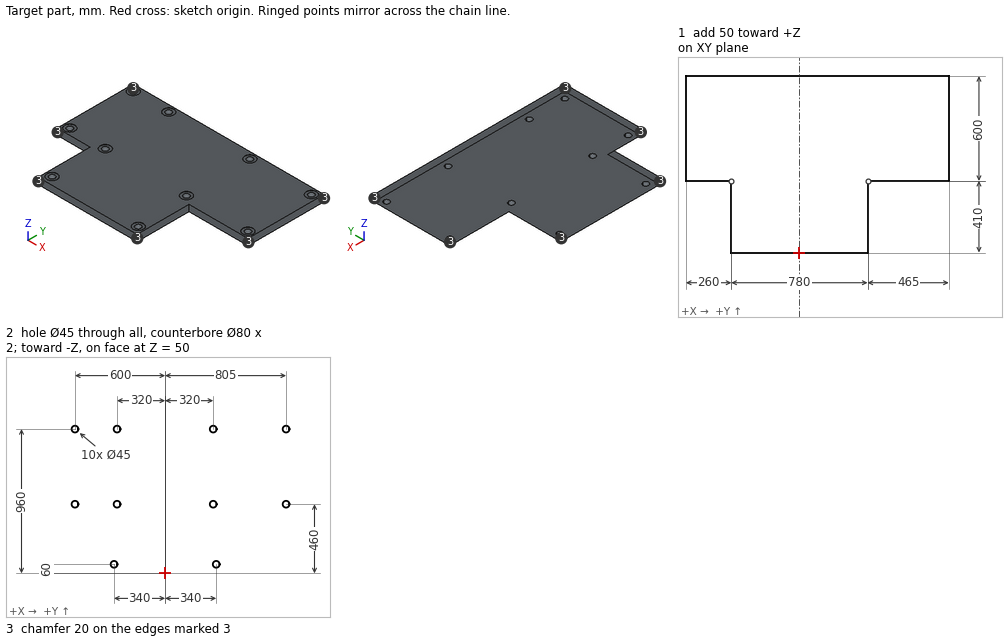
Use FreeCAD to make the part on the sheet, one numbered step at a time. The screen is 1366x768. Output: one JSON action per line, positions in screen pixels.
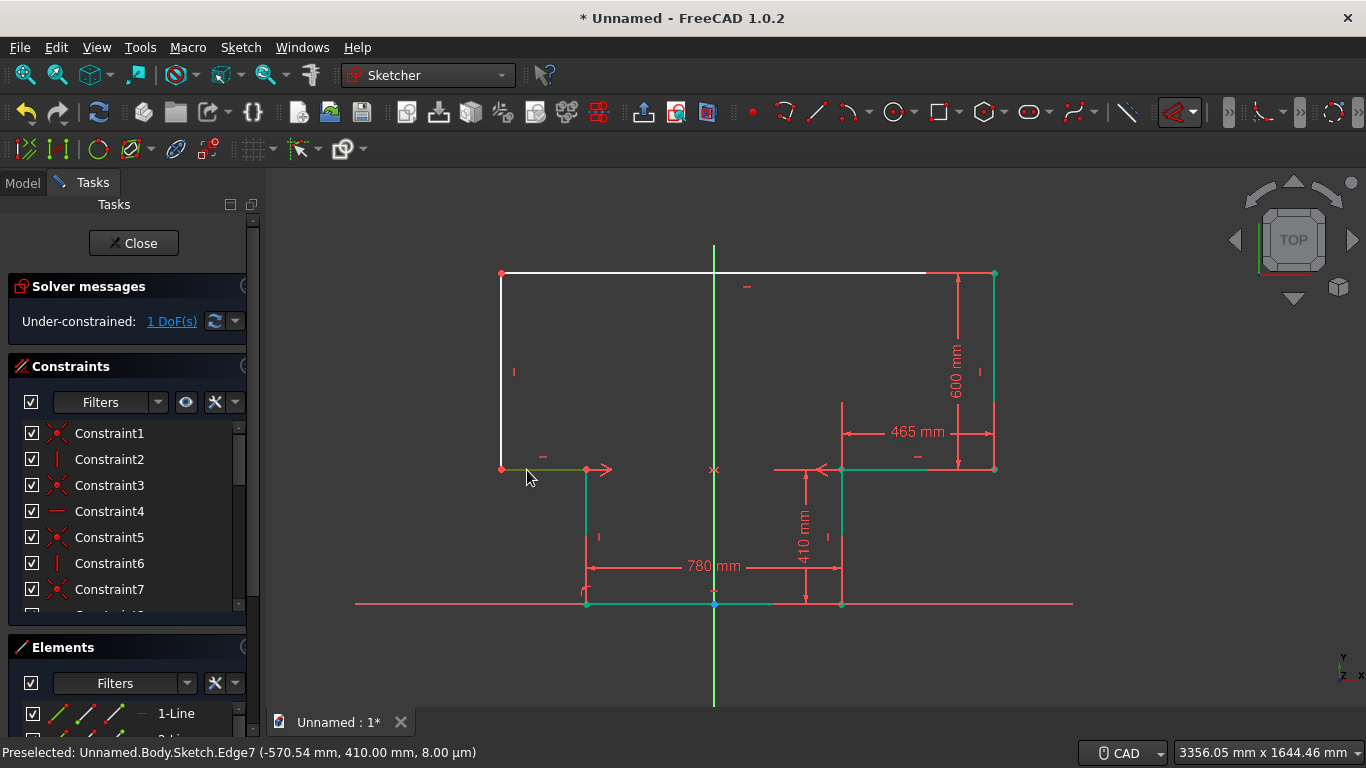
{"action": "key", "text": "l"}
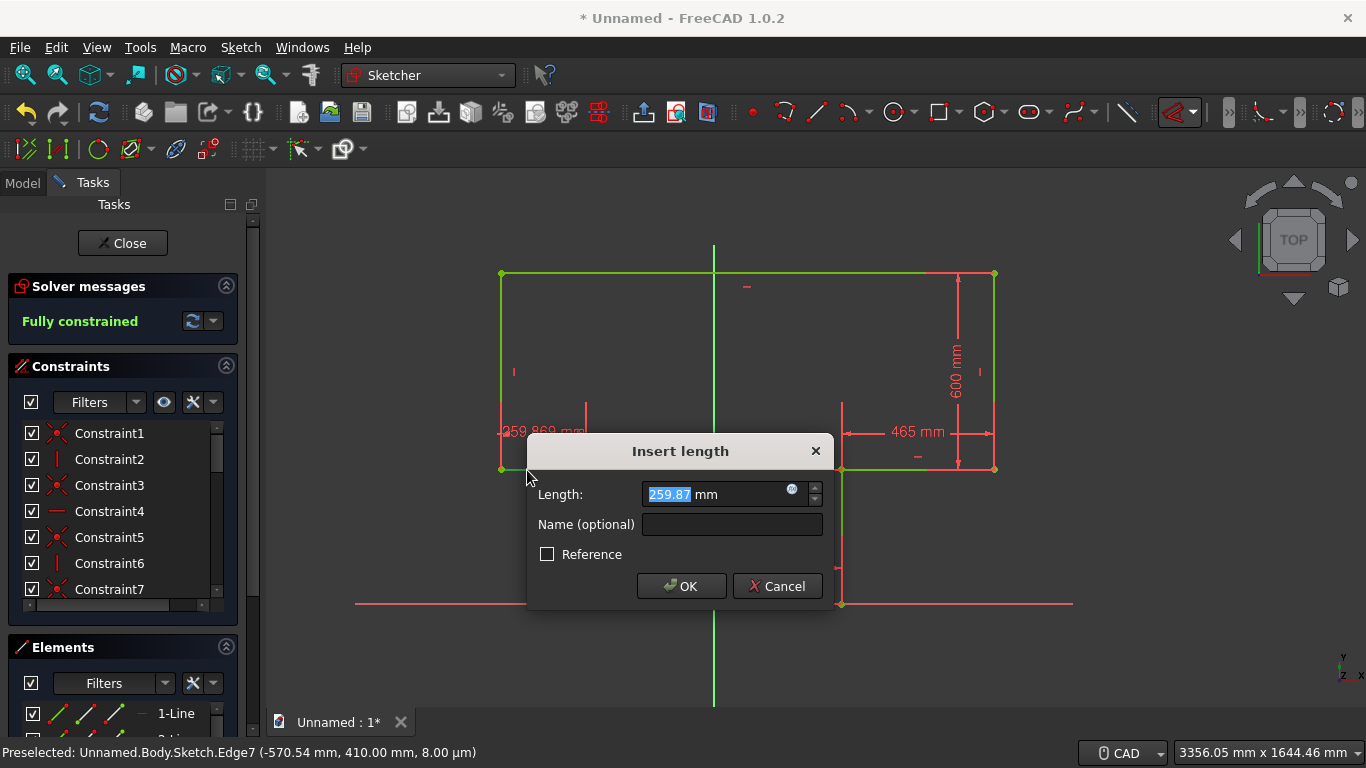
{"action": "type", "text": "260"}
{"action": "key", "text": "Return"}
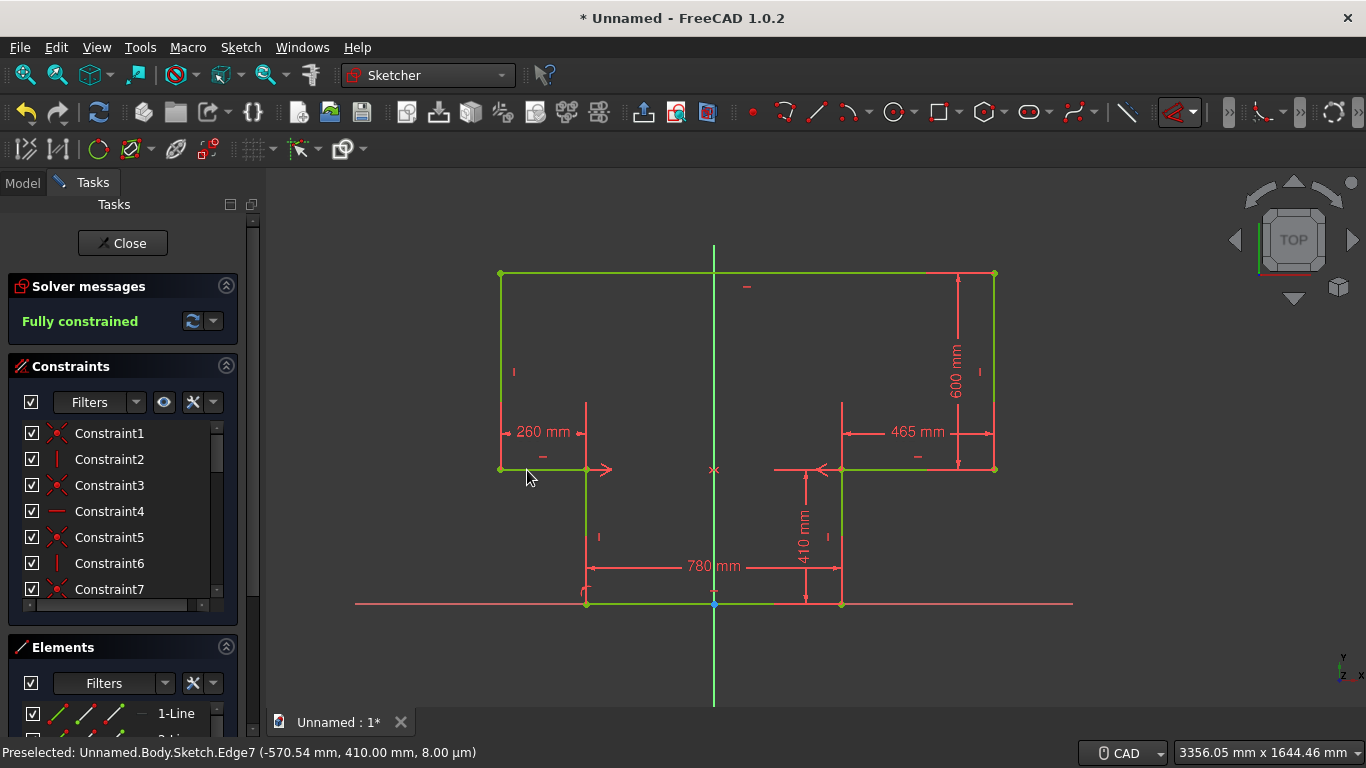
{"action": "left_click", "coordinate": [123, 243]}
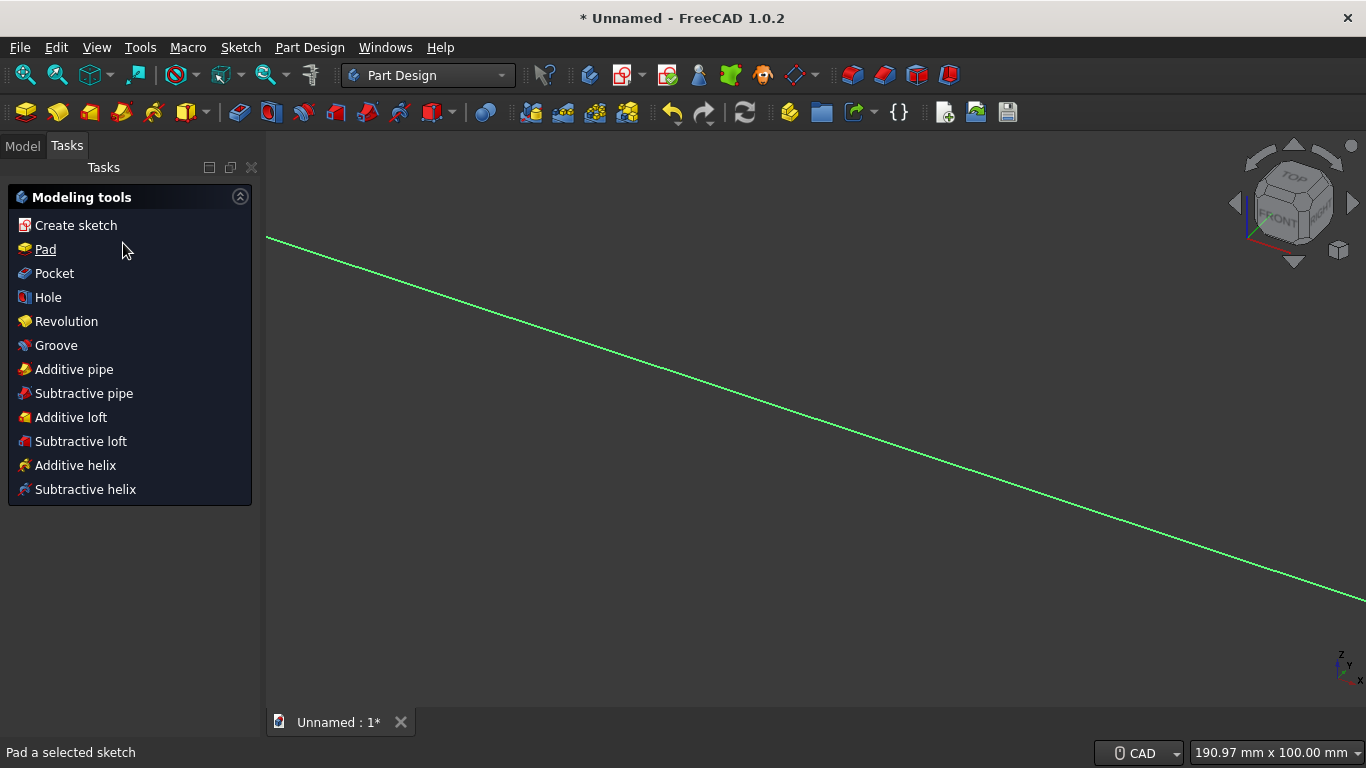
{"action": "left_click", "coordinate": [26, 112]}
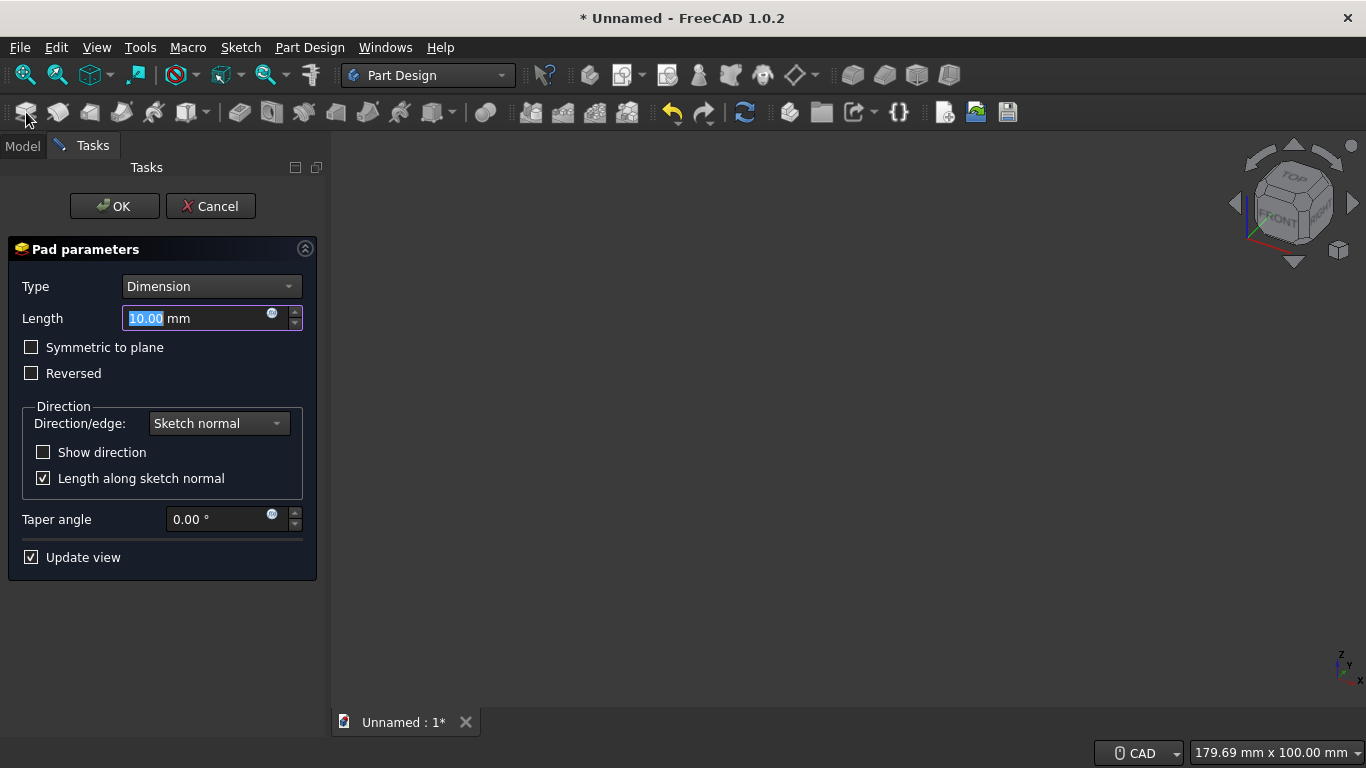
{"action": "type", "text": "50"}
{"action": "key", "text": "Tab"}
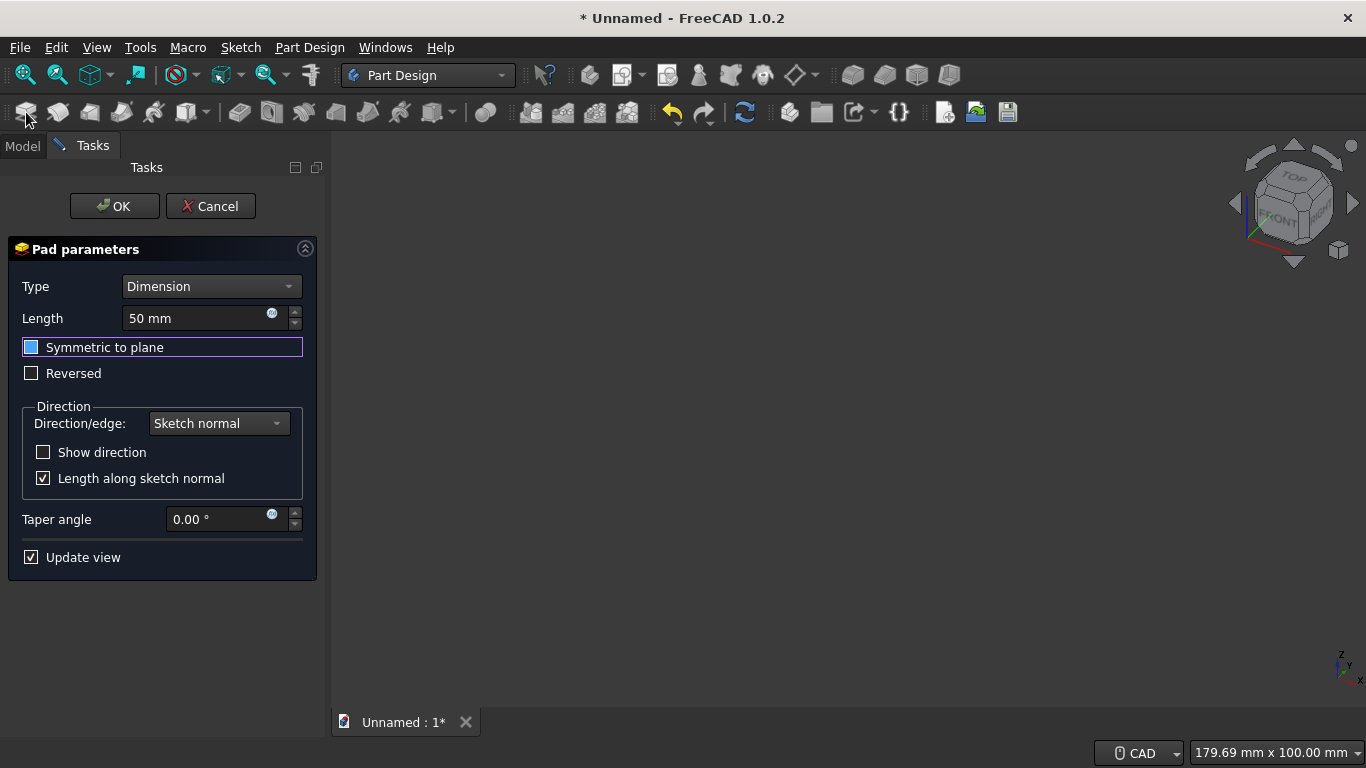
{"action": "left_click", "coordinate": [115, 206]}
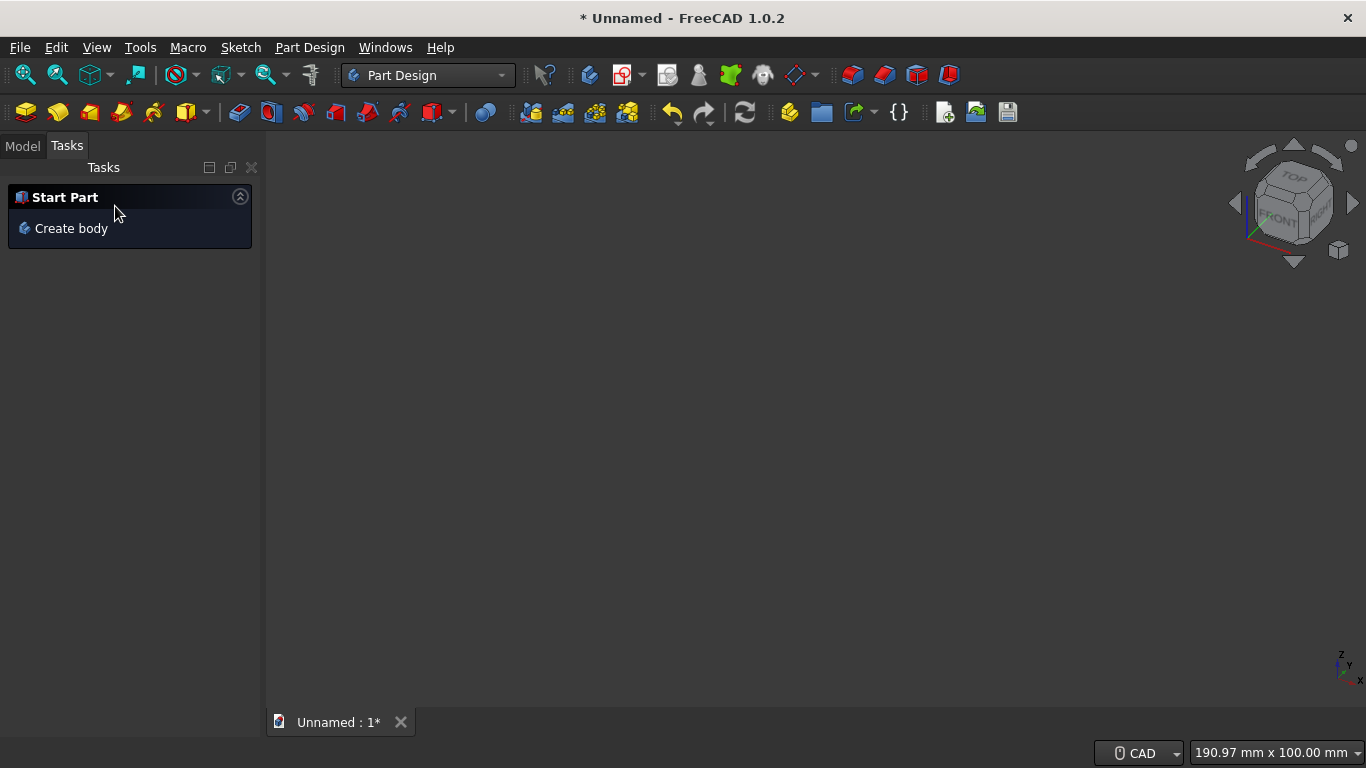
{"action": "key", "text": "v f"}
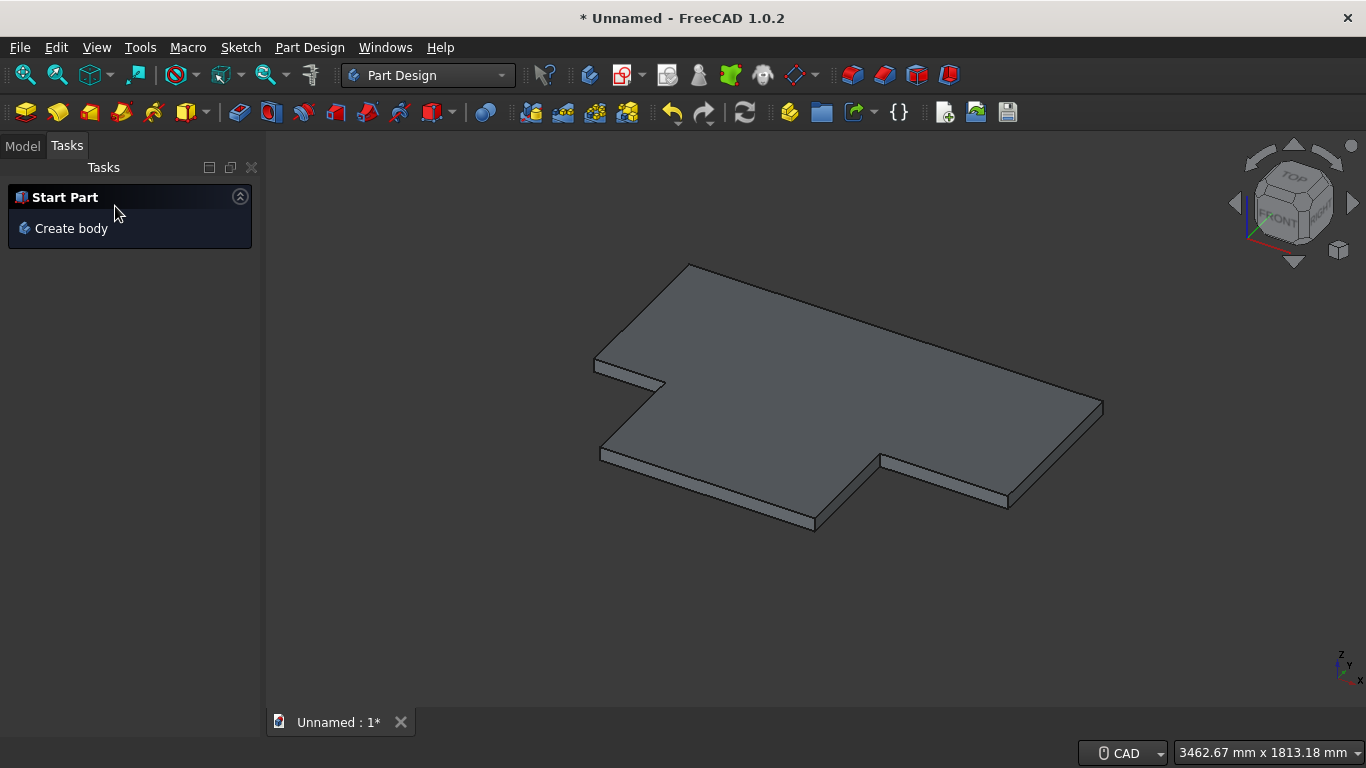
{"action": "left_click", "coordinate": [839, 389]}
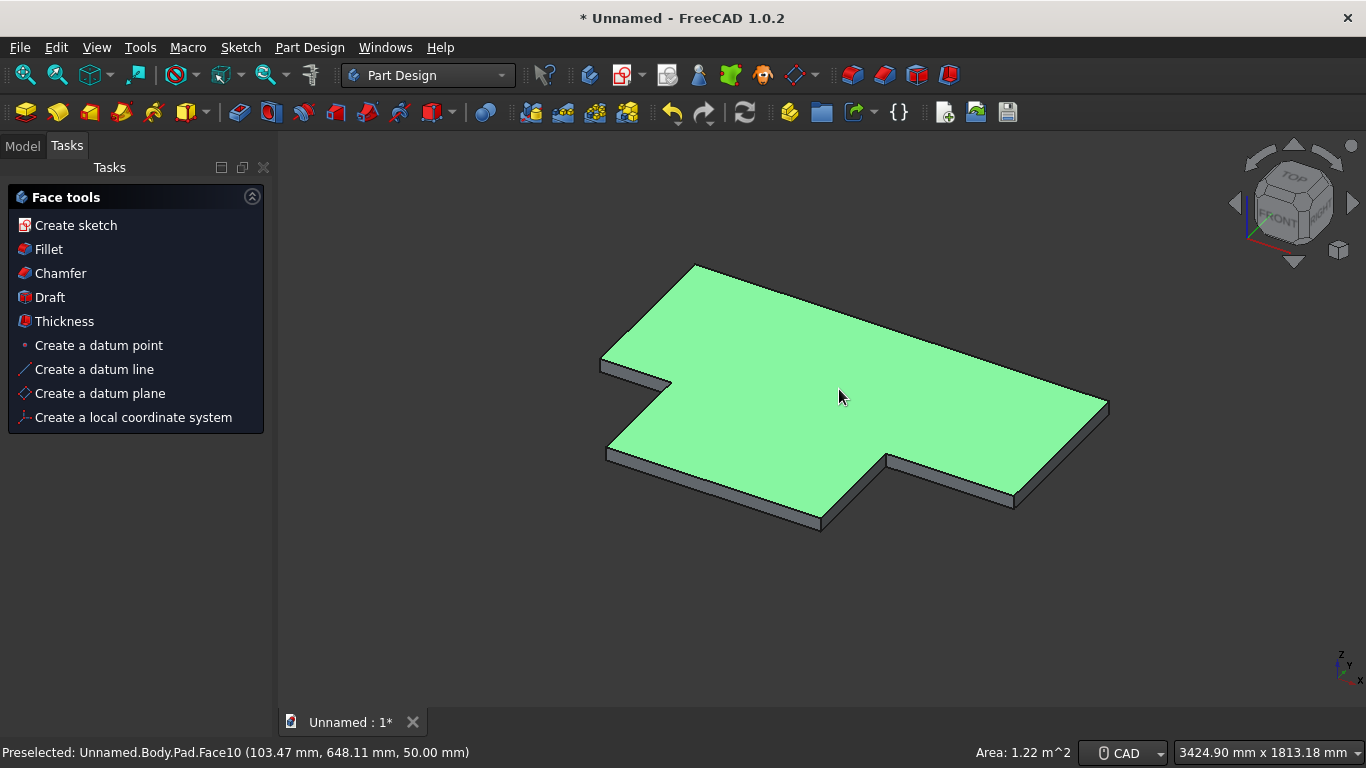
{"action": "left_click", "coordinate": [622, 76]}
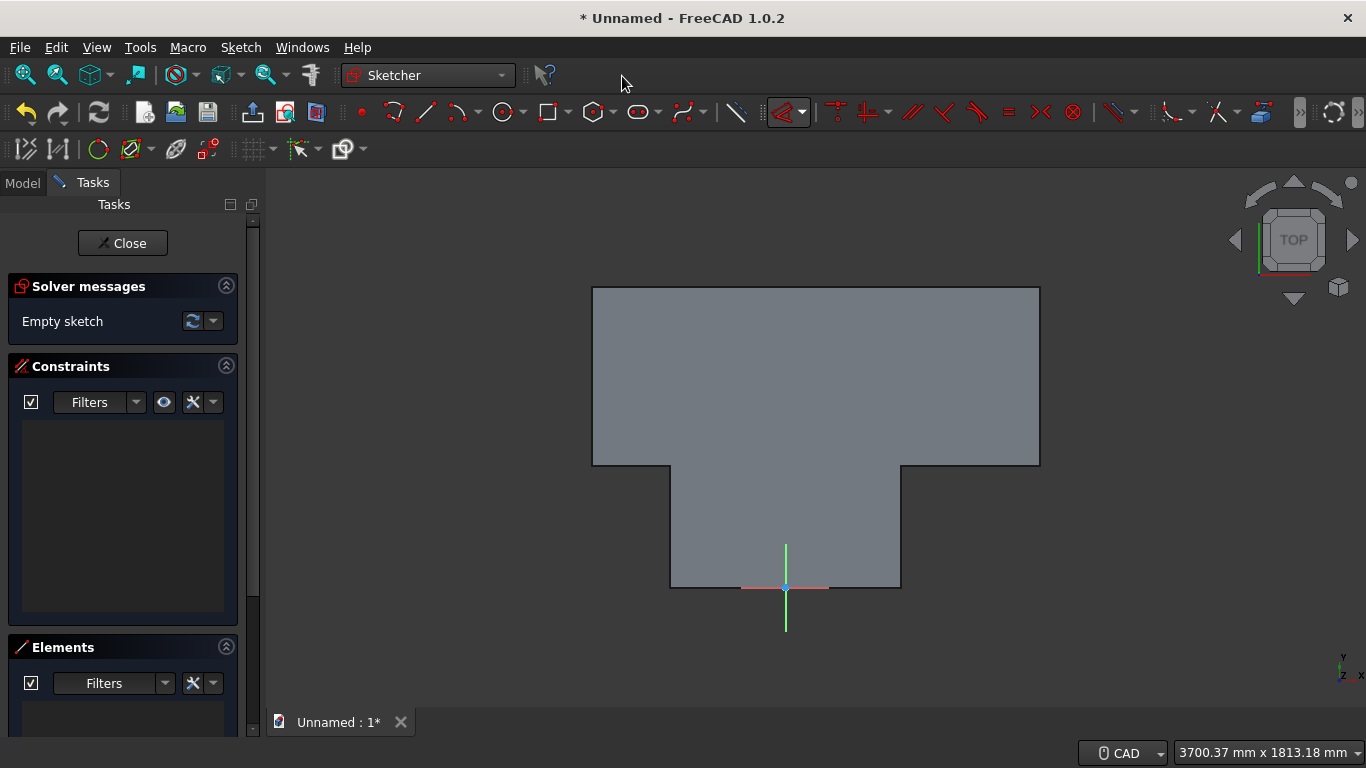
{"action": "left_click", "coordinate": [504, 112]}